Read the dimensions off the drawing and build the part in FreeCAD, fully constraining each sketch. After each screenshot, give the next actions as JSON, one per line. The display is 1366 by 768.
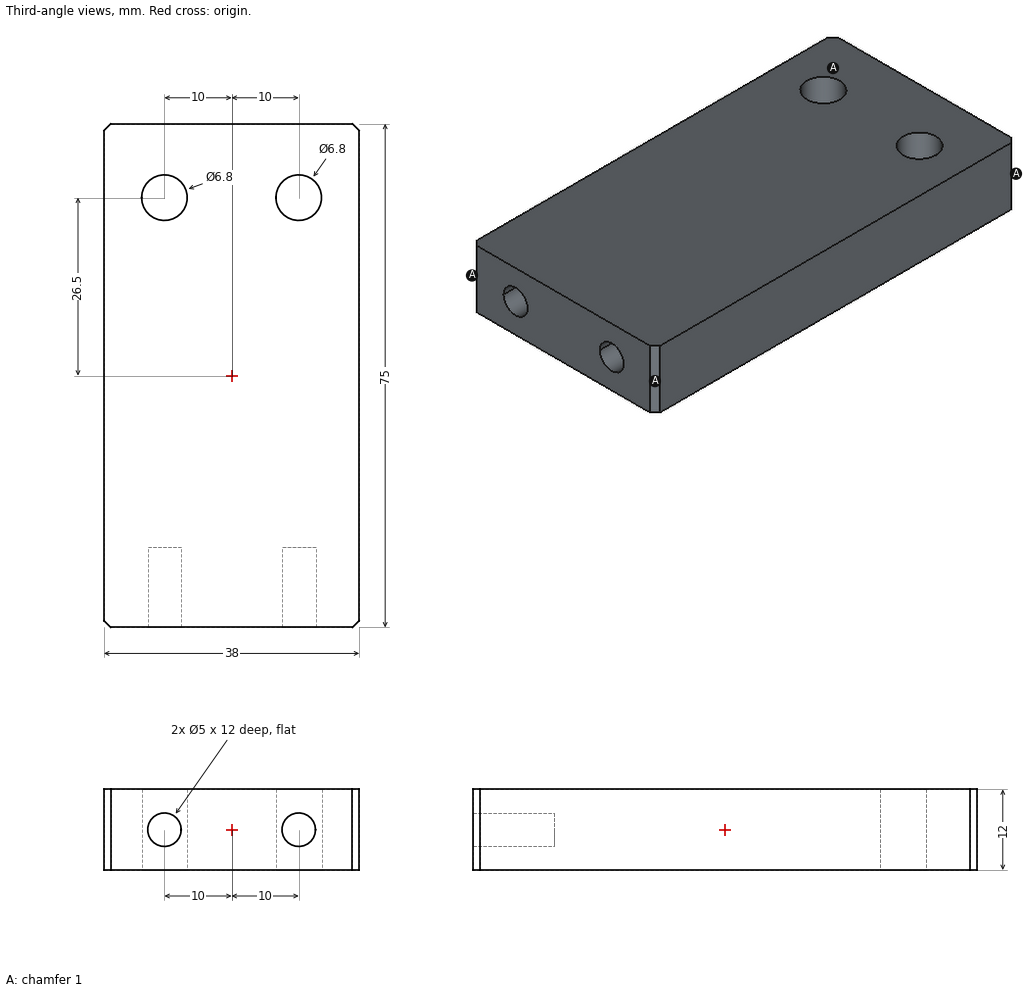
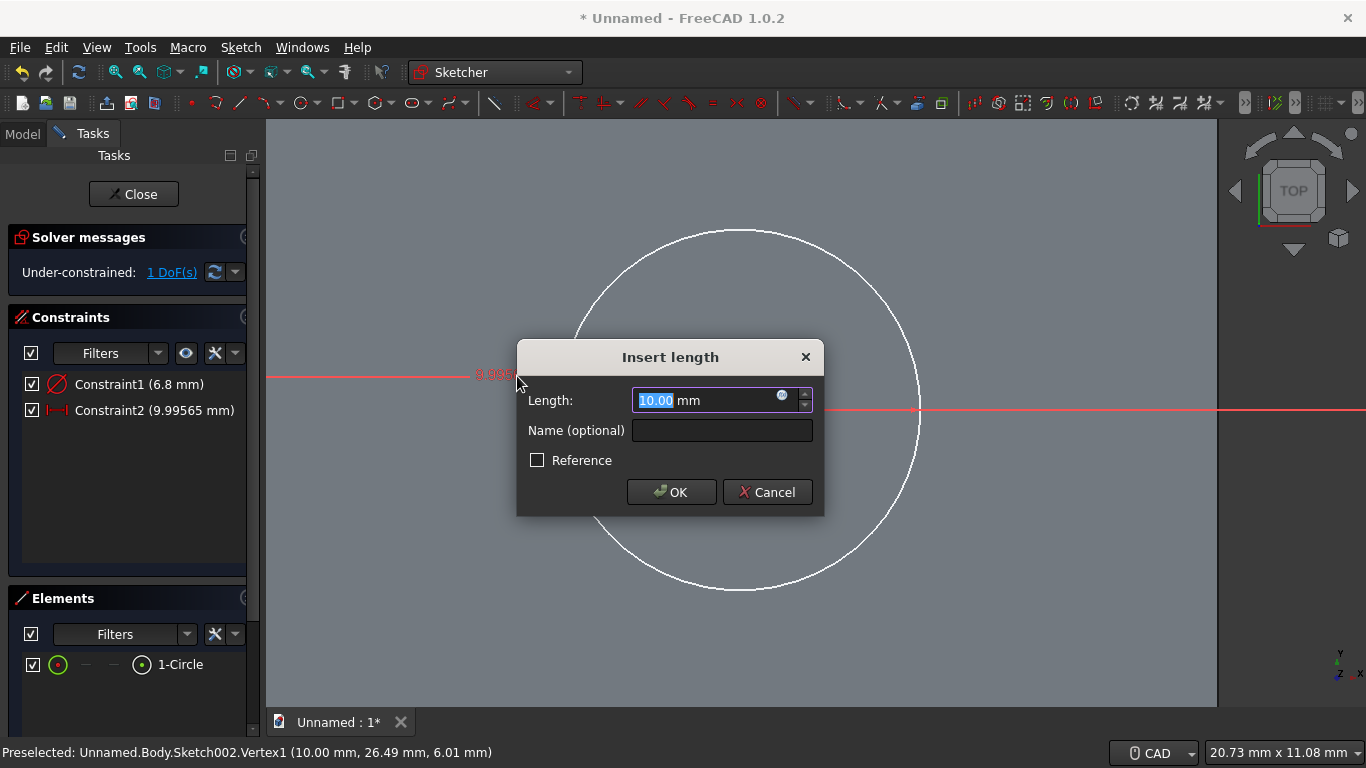
{"action": "type", "text": "10"}
{"action": "key", "text": "Return"}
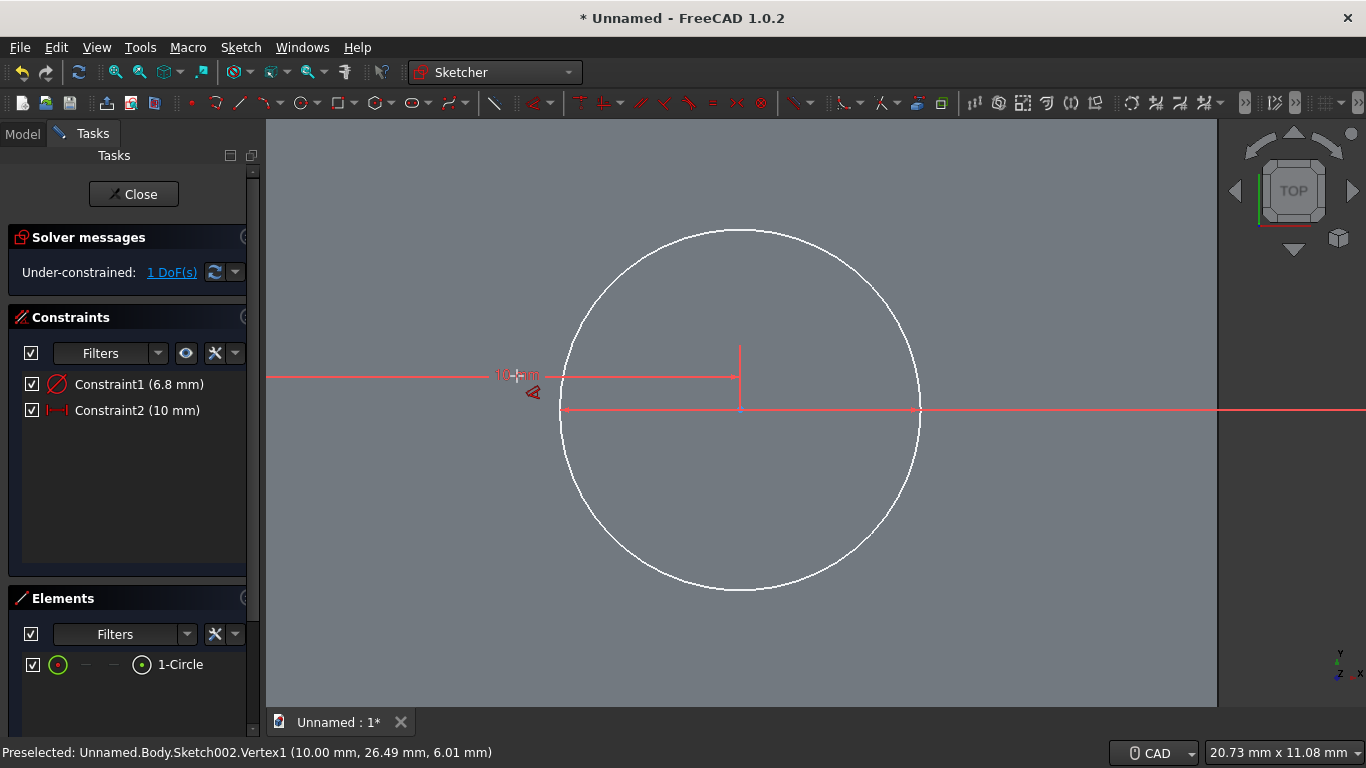
{"action": "left_click", "coordinate": [740, 410]}
{"action": "left_click", "coordinate": [774, 545]}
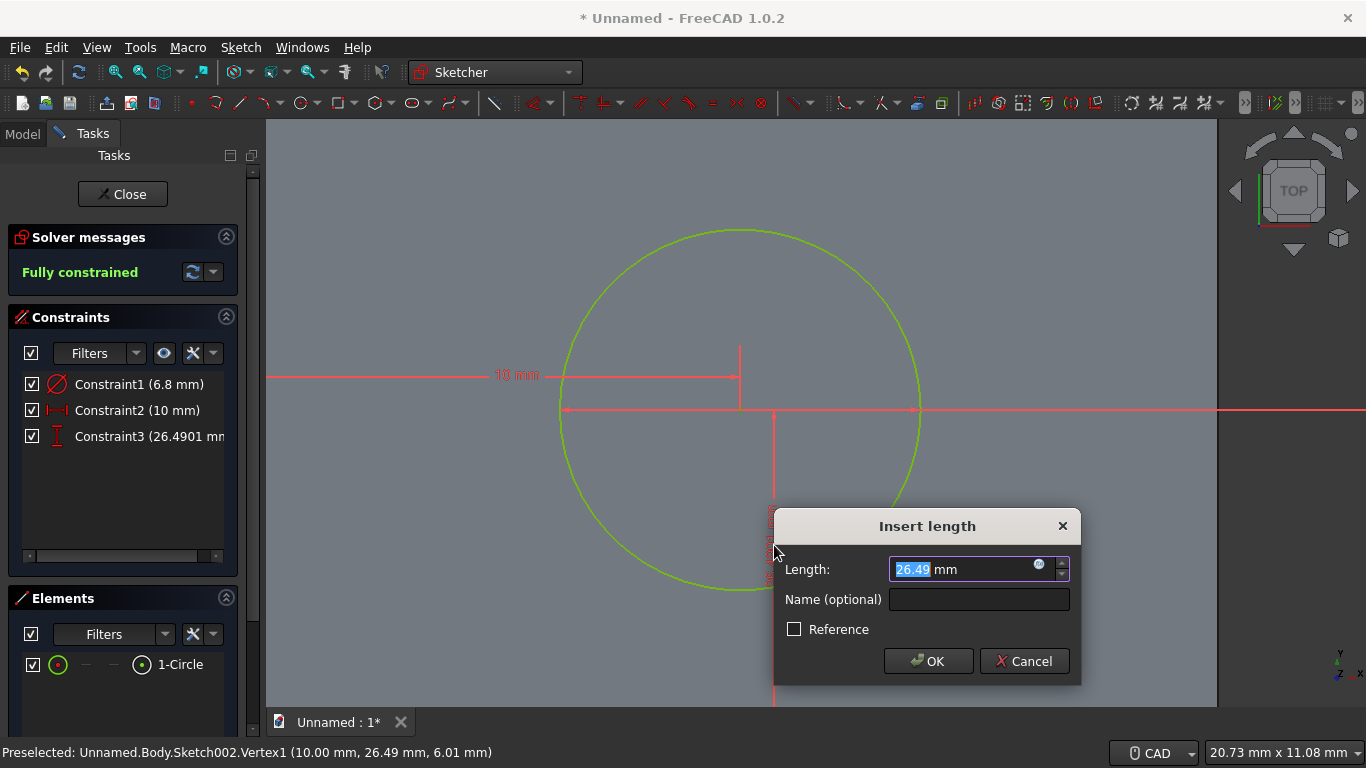
{"action": "type", "text": "26.5"}
{"action": "key", "text": "Return"}
{"action": "key", "text": "Escape"}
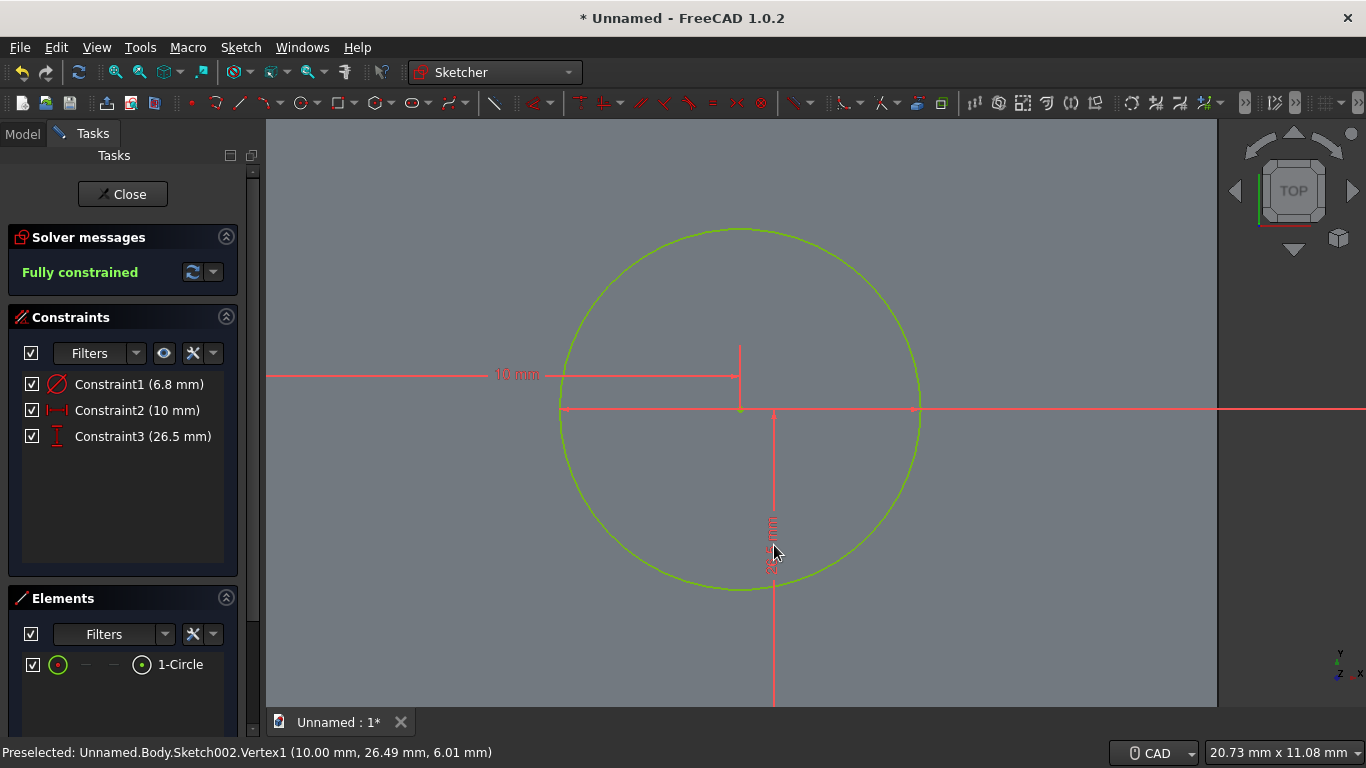
{"action": "left_click", "coordinate": [123, 194]}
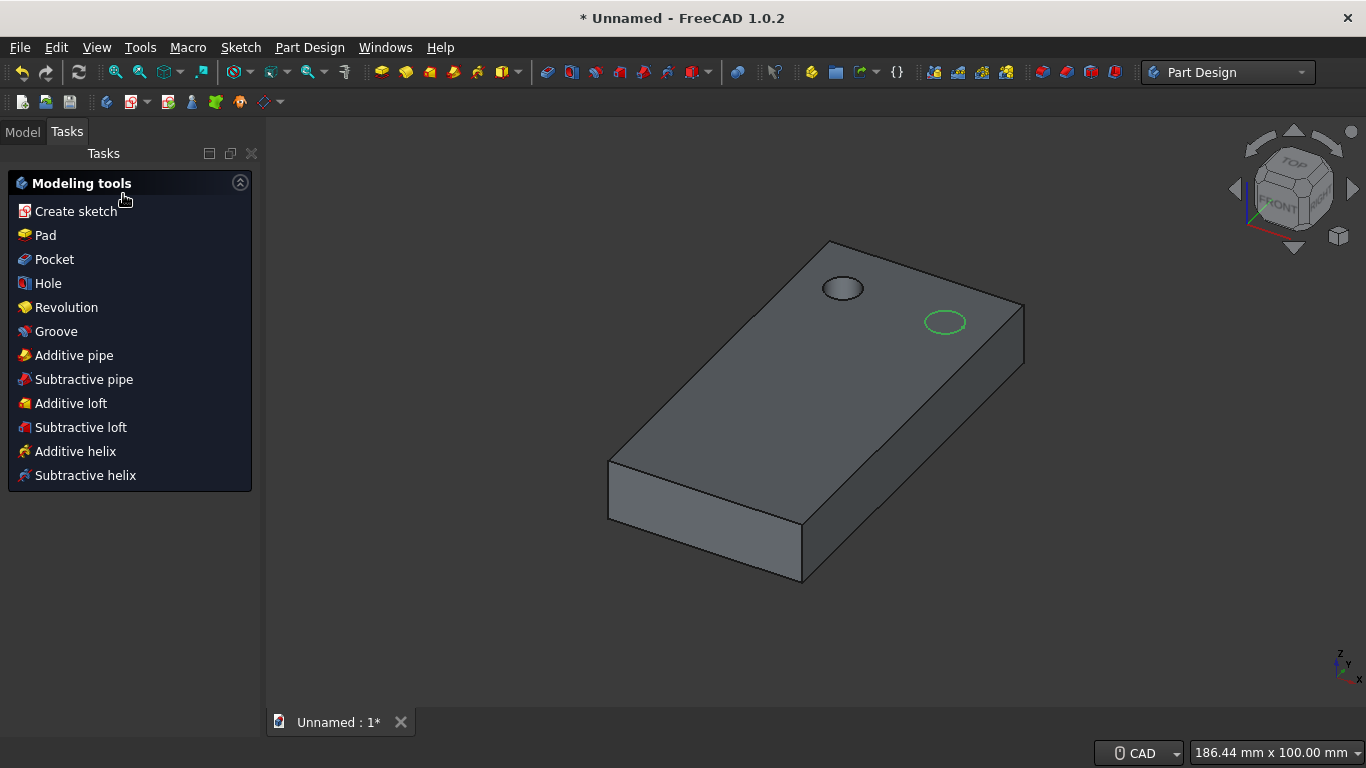
{"action": "left_click", "coordinate": [548, 72]}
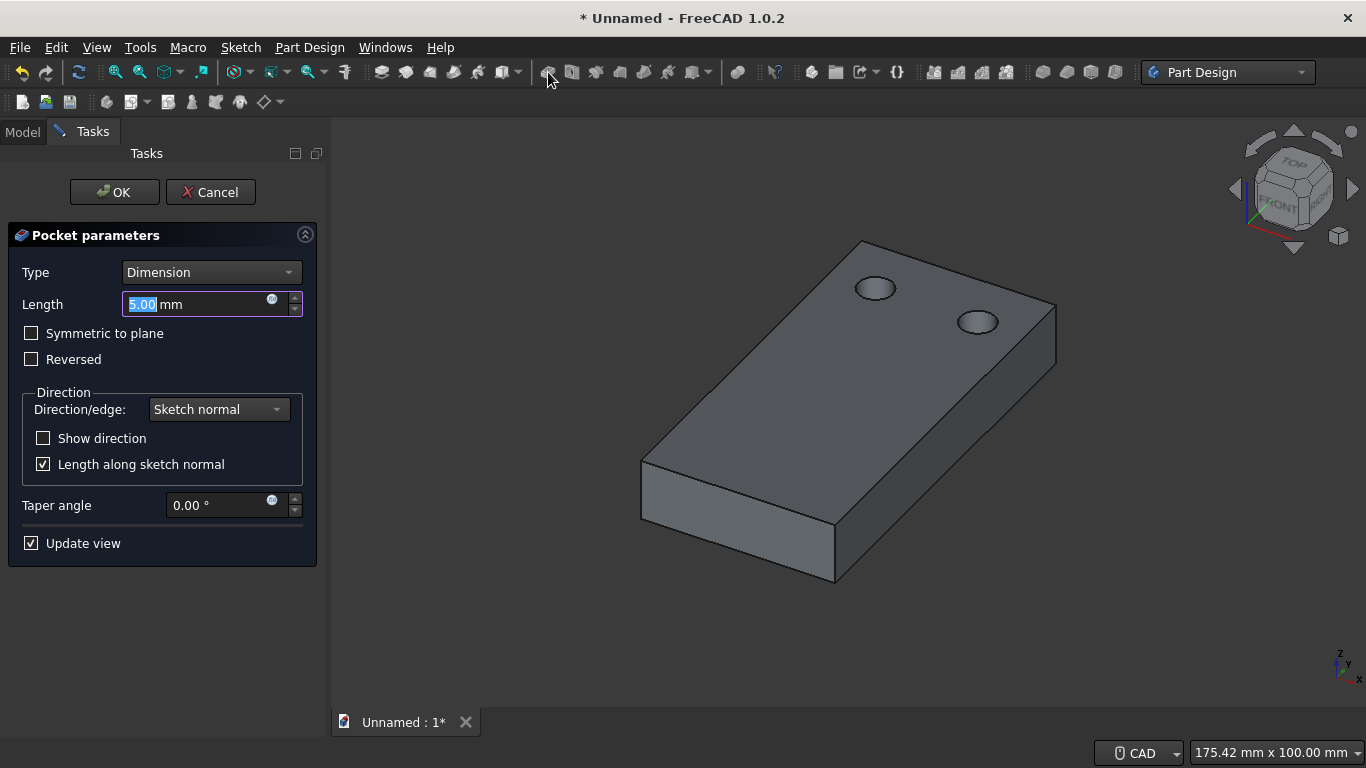
{"action": "left_click", "coordinate": [212, 272]}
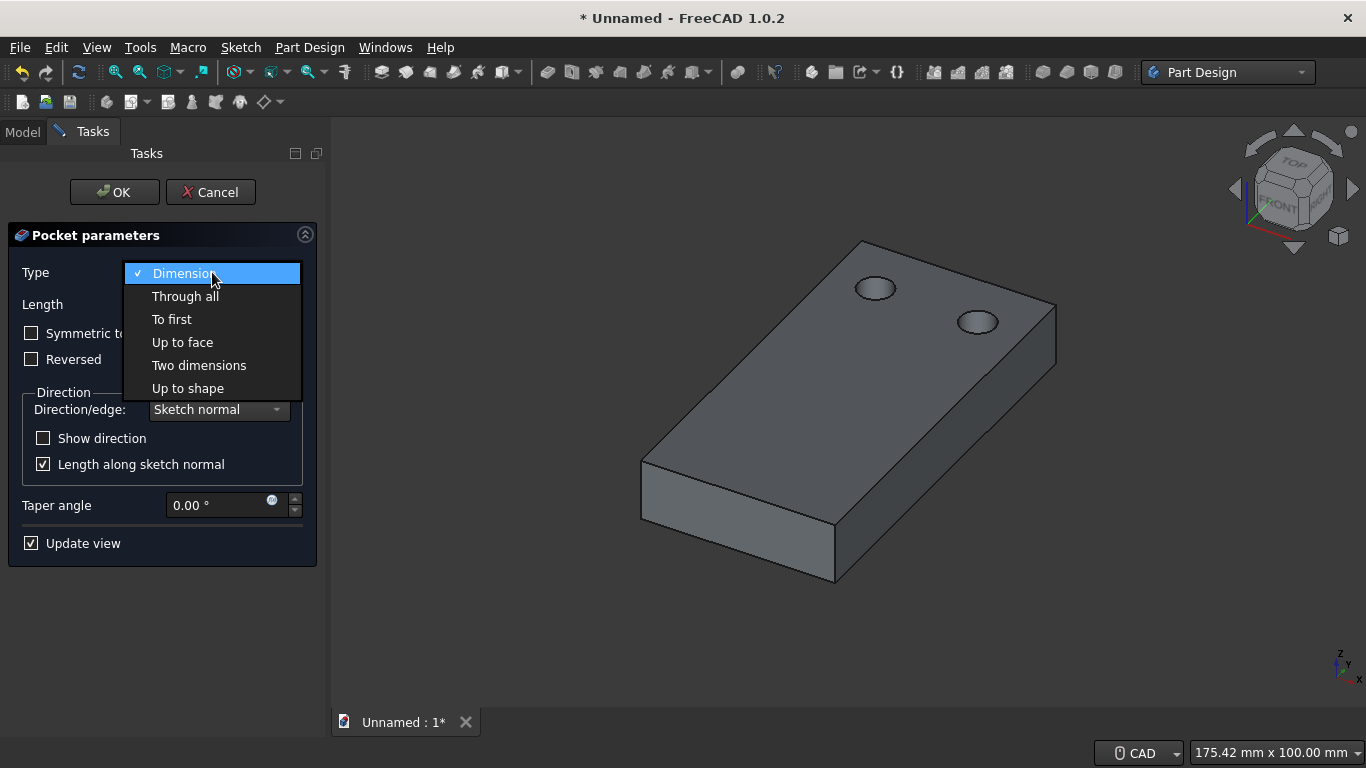
{"action": "left_click", "coordinate": [212, 296]}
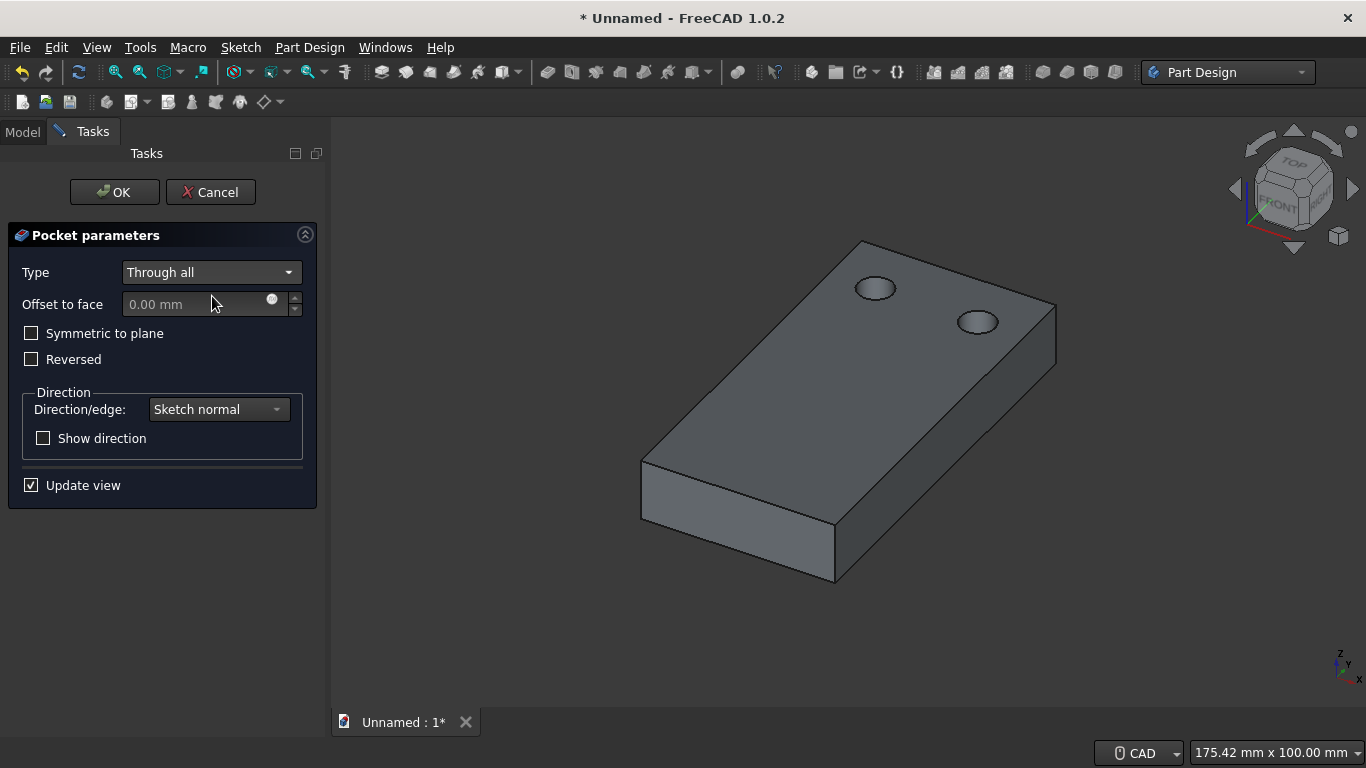
{"action": "left_click", "coordinate": [115, 192]}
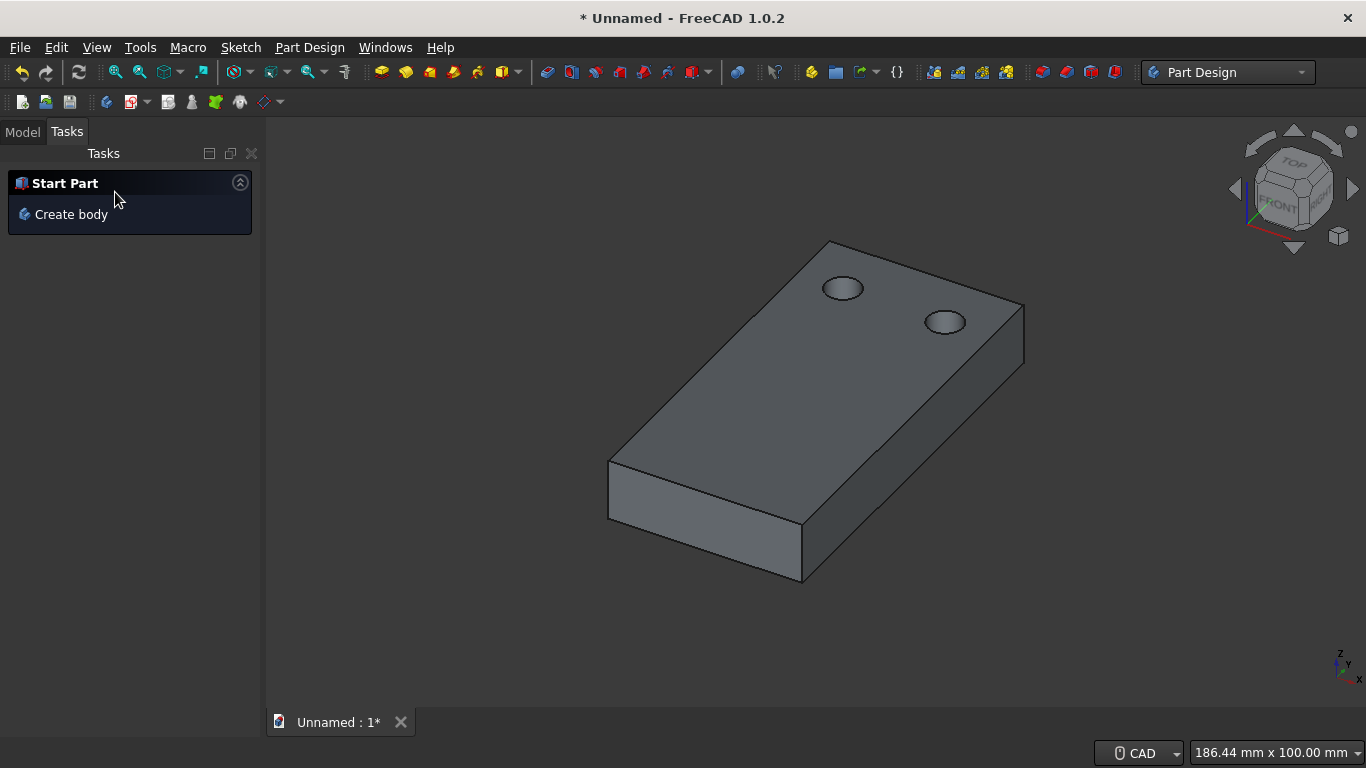
{"action": "left_click", "coordinate": [761, 539]}